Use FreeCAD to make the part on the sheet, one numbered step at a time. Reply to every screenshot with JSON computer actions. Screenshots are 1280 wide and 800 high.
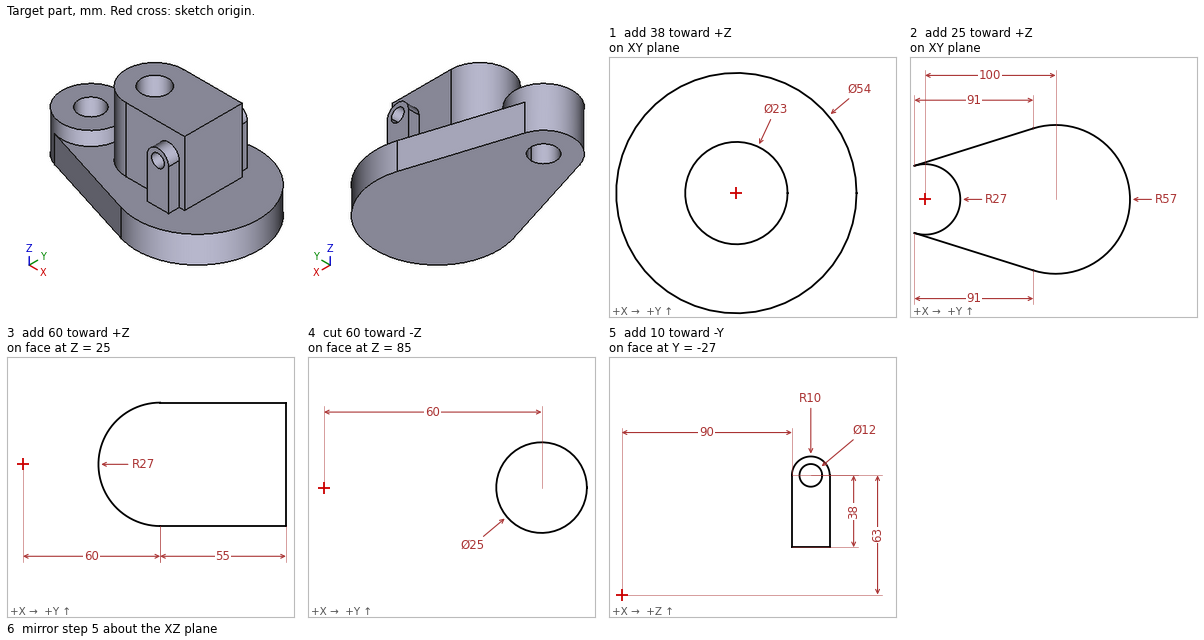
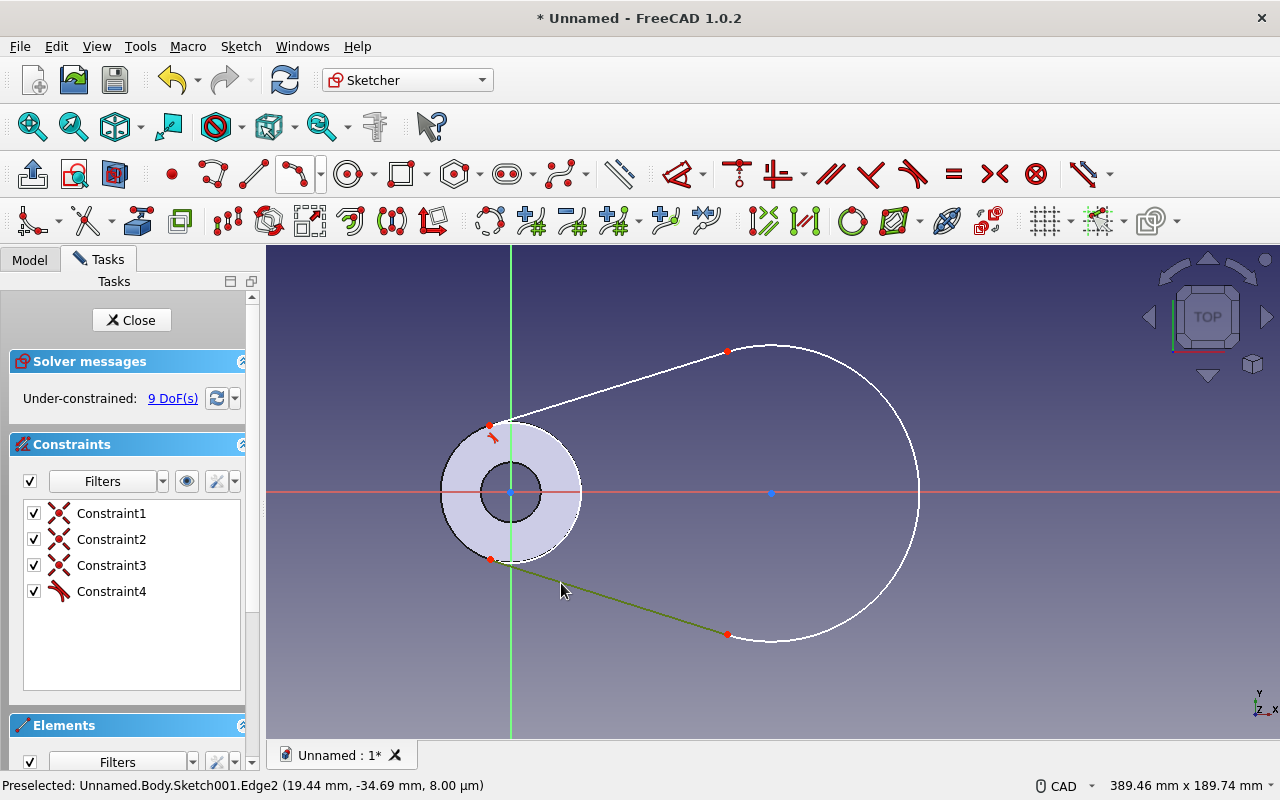
{"action": "left_click", "coordinate": [562, 541]}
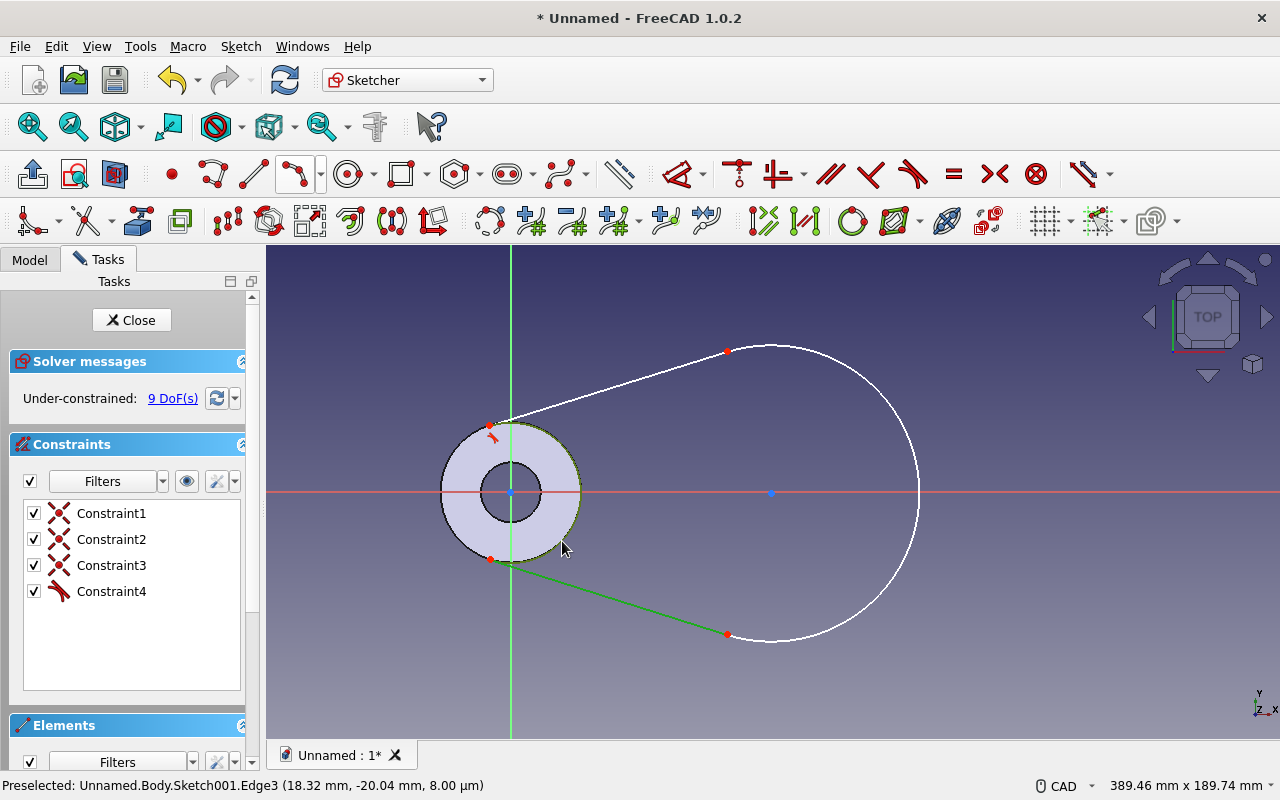
{"action": "key", "text": "t"}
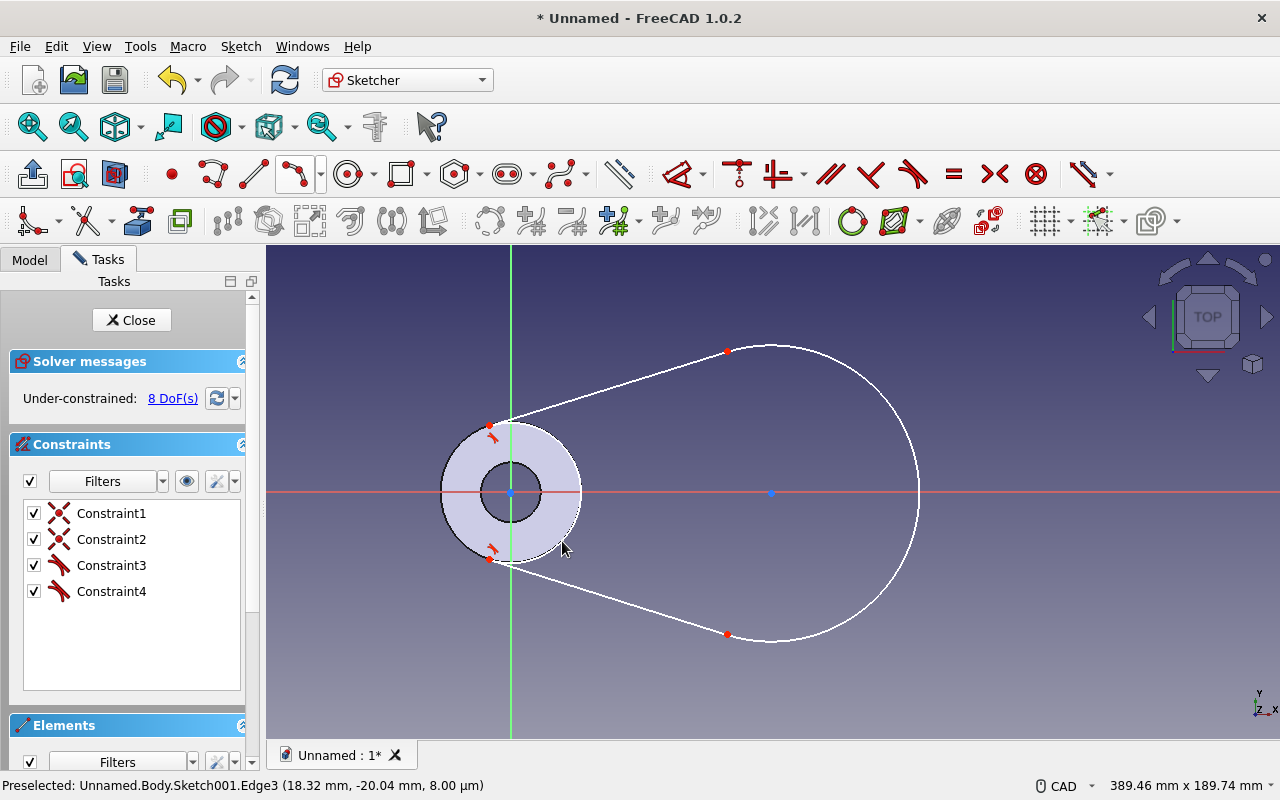
{"action": "left_click_drag", "start_coordinate": [501, 482], "coordinate": [521, 503]}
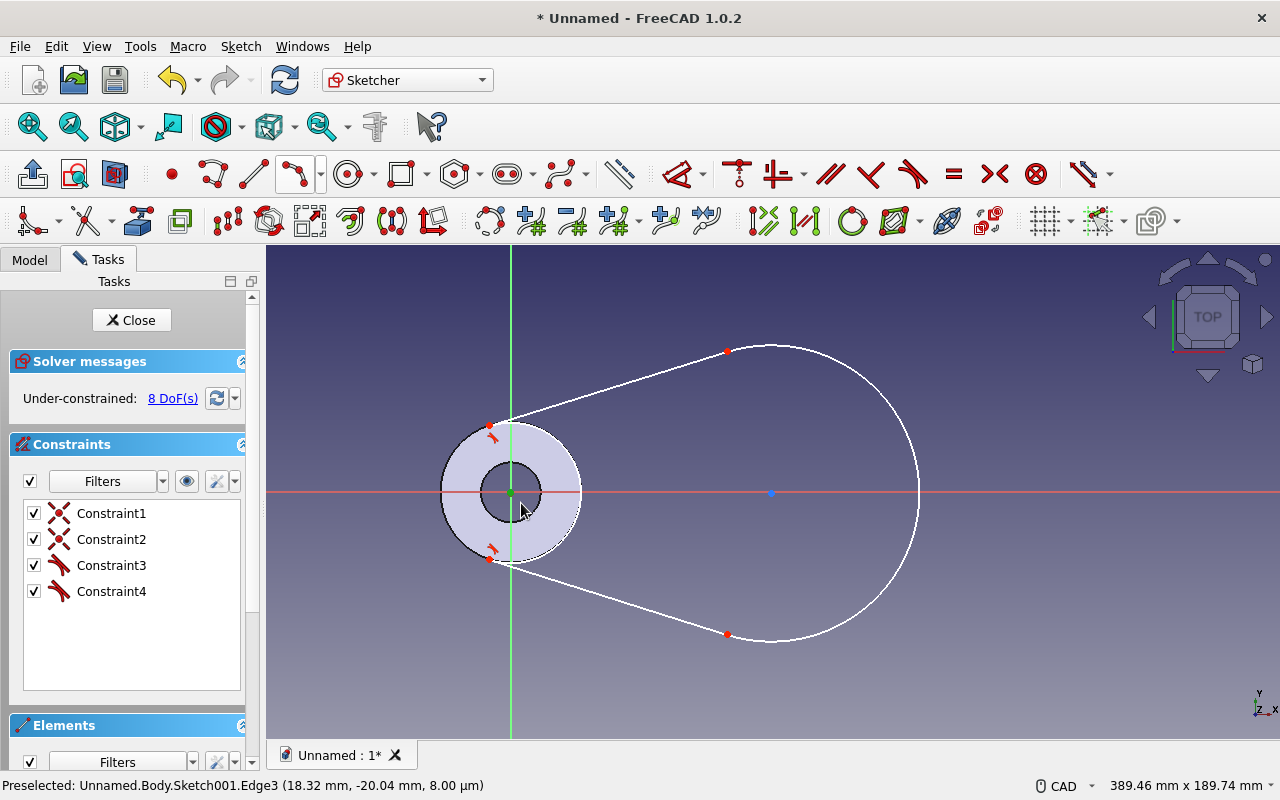
{"action": "key", "text": "c"}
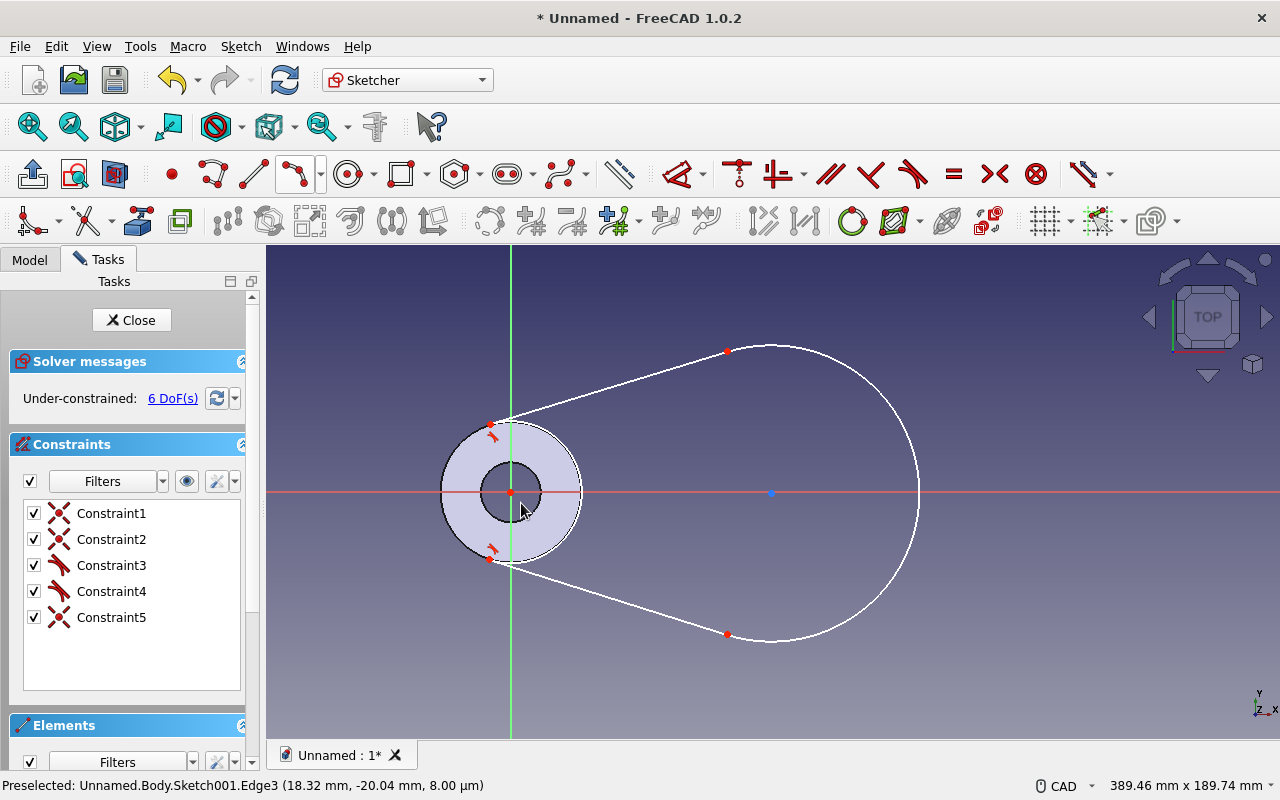
{"action": "left_click", "coordinate": [771, 493]}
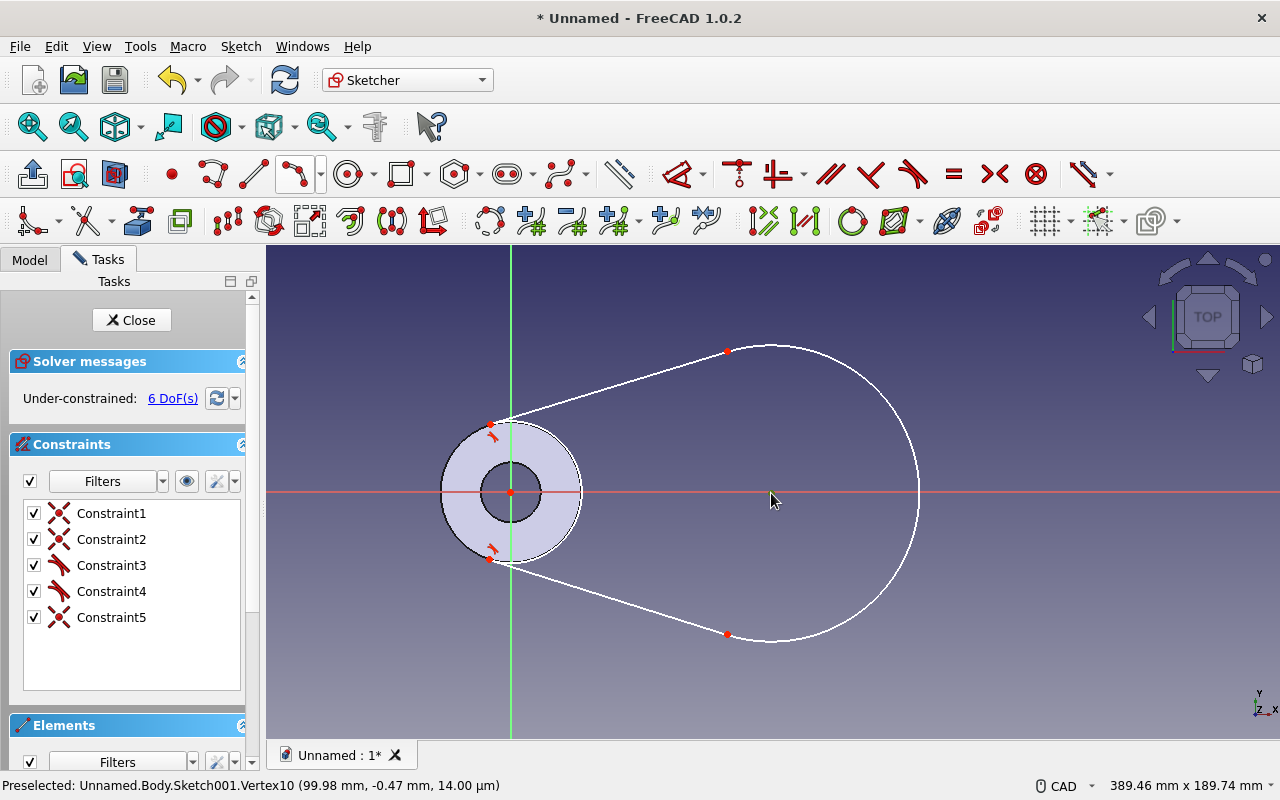
{"action": "left_click", "coordinate": [353, 492]}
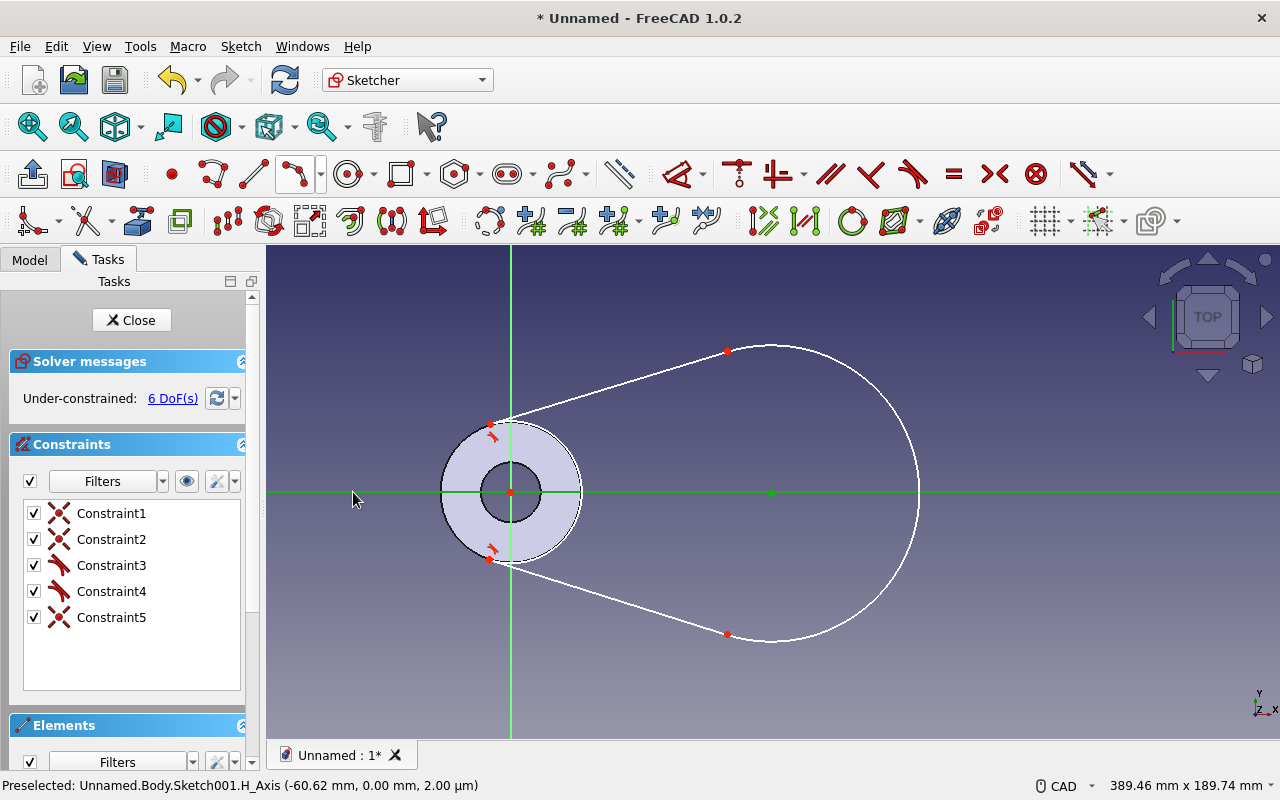
{"action": "key", "text": "c"}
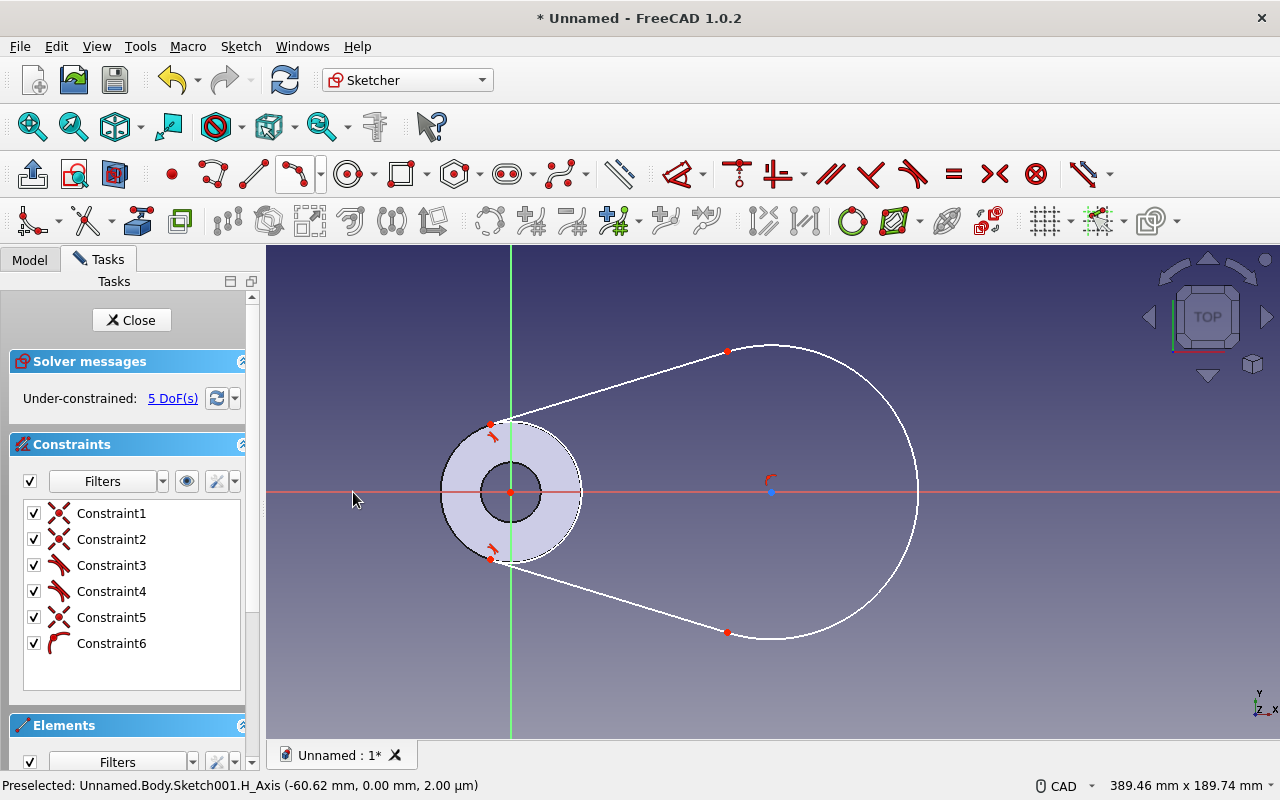
{"action": "key", "text": "d"}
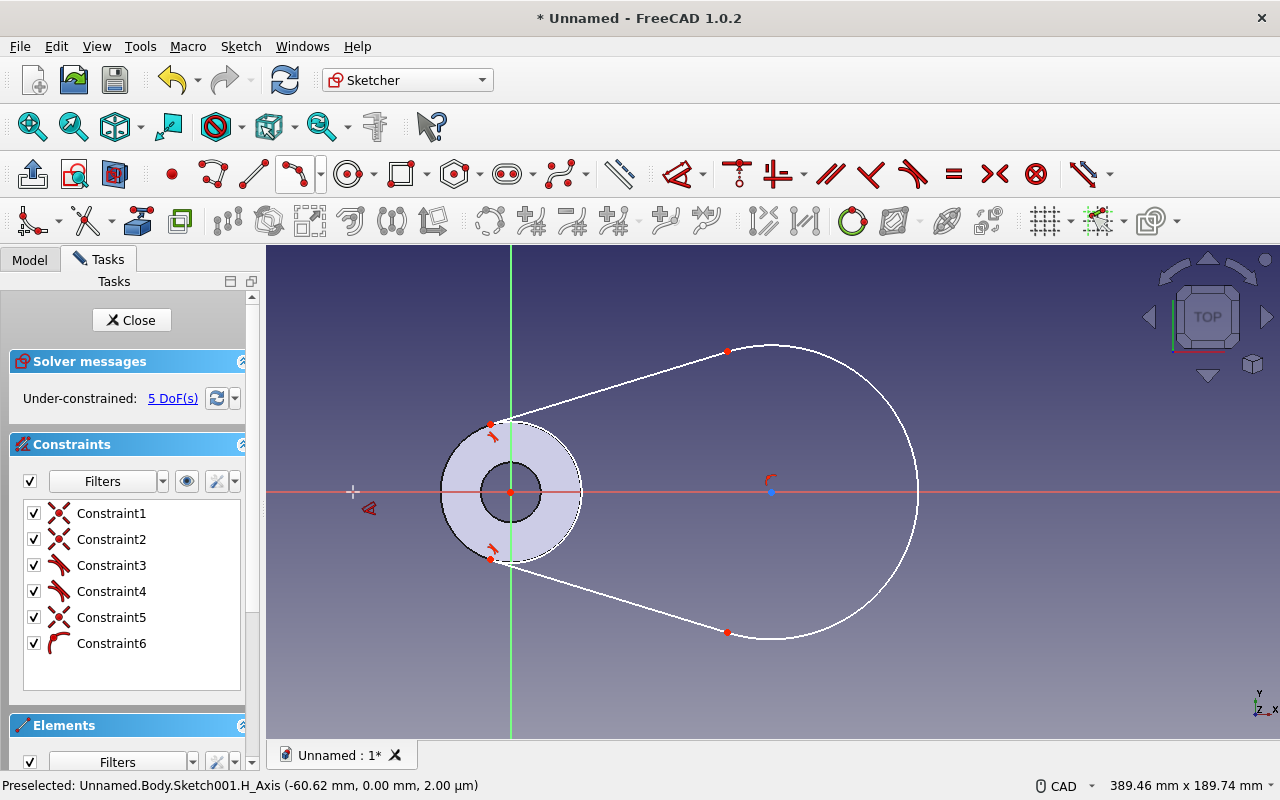
{"action": "left_click", "coordinate": [563, 540]}
{"action": "left_click", "coordinate": [587, 562]}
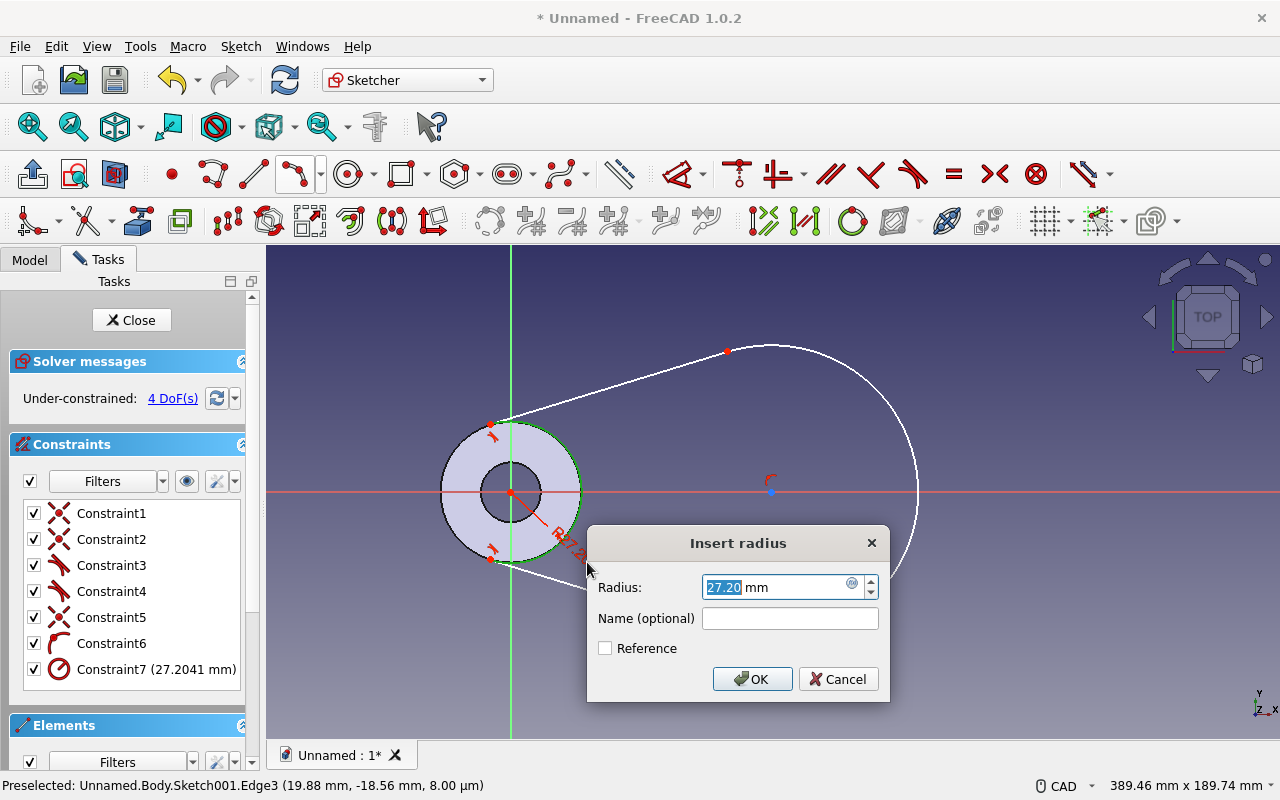
{"action": "type", "text": "27"}
{"action": "key", "text": "Return"}